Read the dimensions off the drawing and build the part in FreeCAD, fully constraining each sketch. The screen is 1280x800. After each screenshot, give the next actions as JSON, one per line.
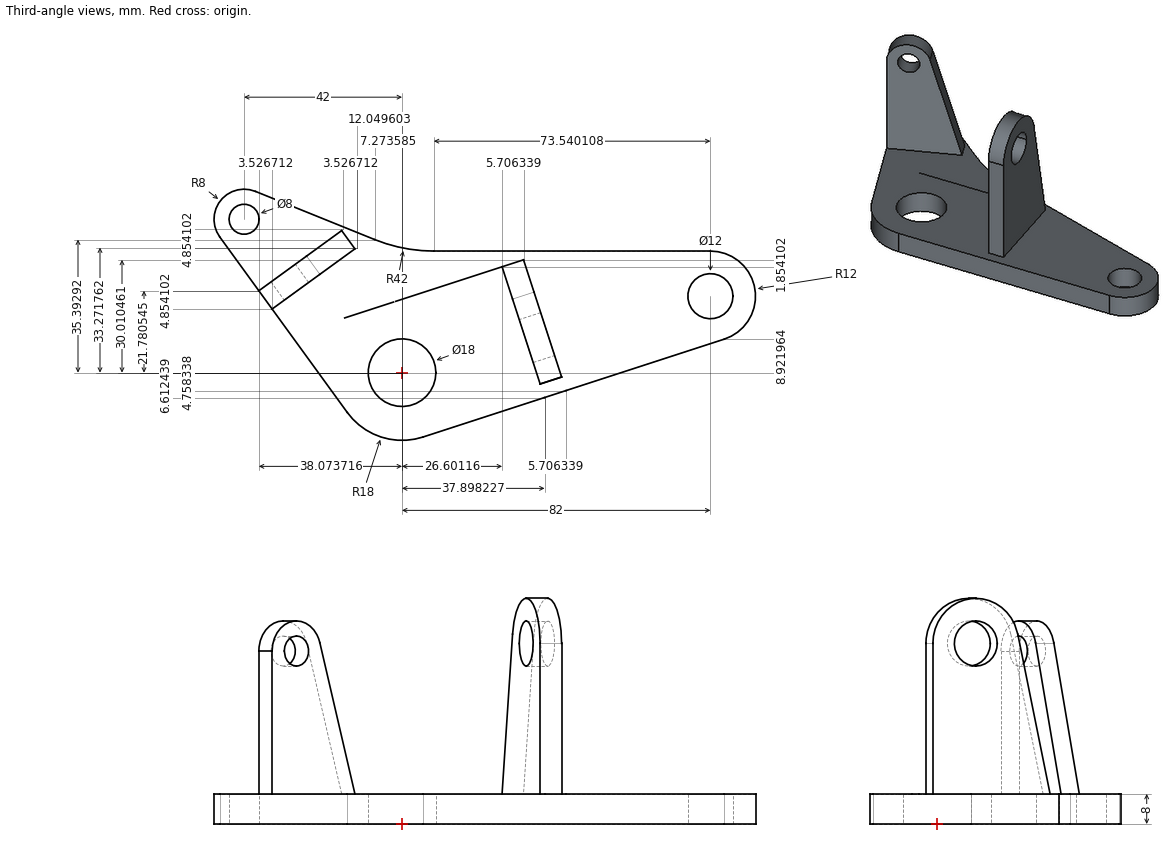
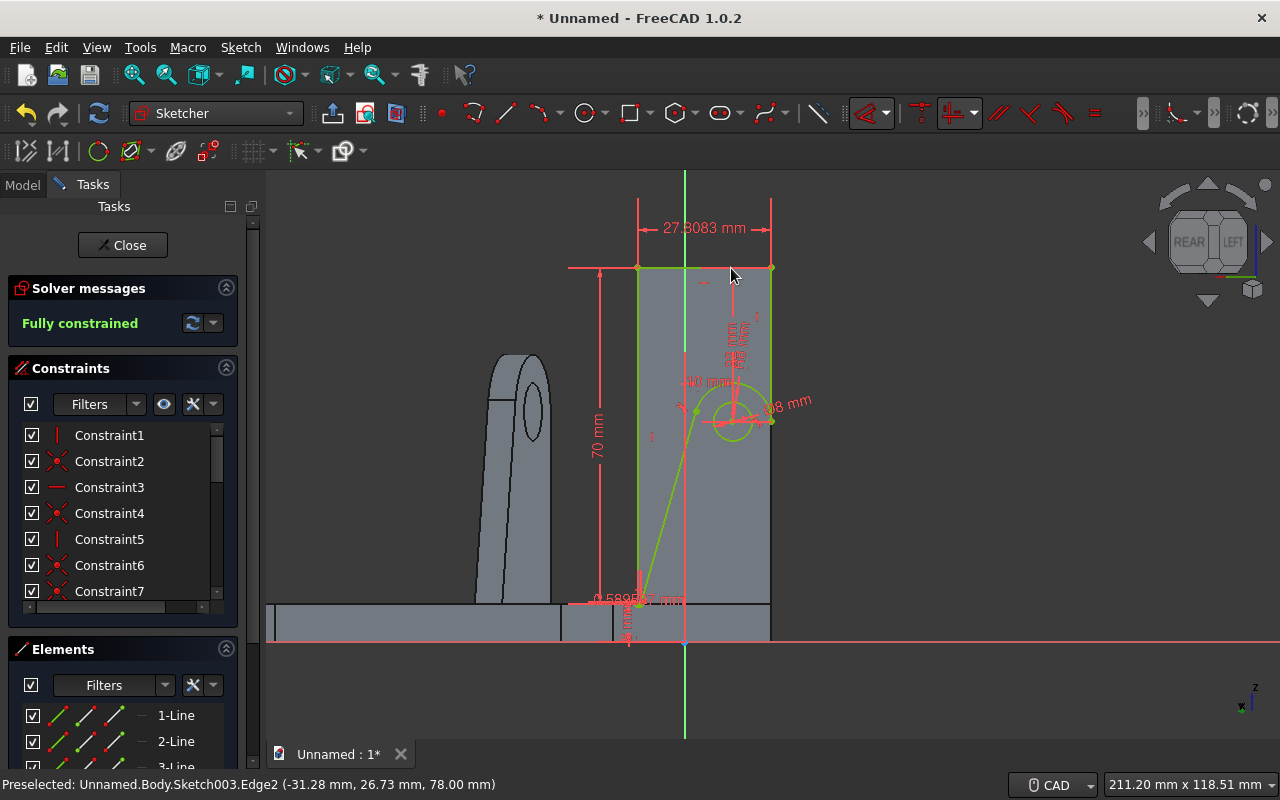
{"action": "left_click", "coordinate": [123, 245]}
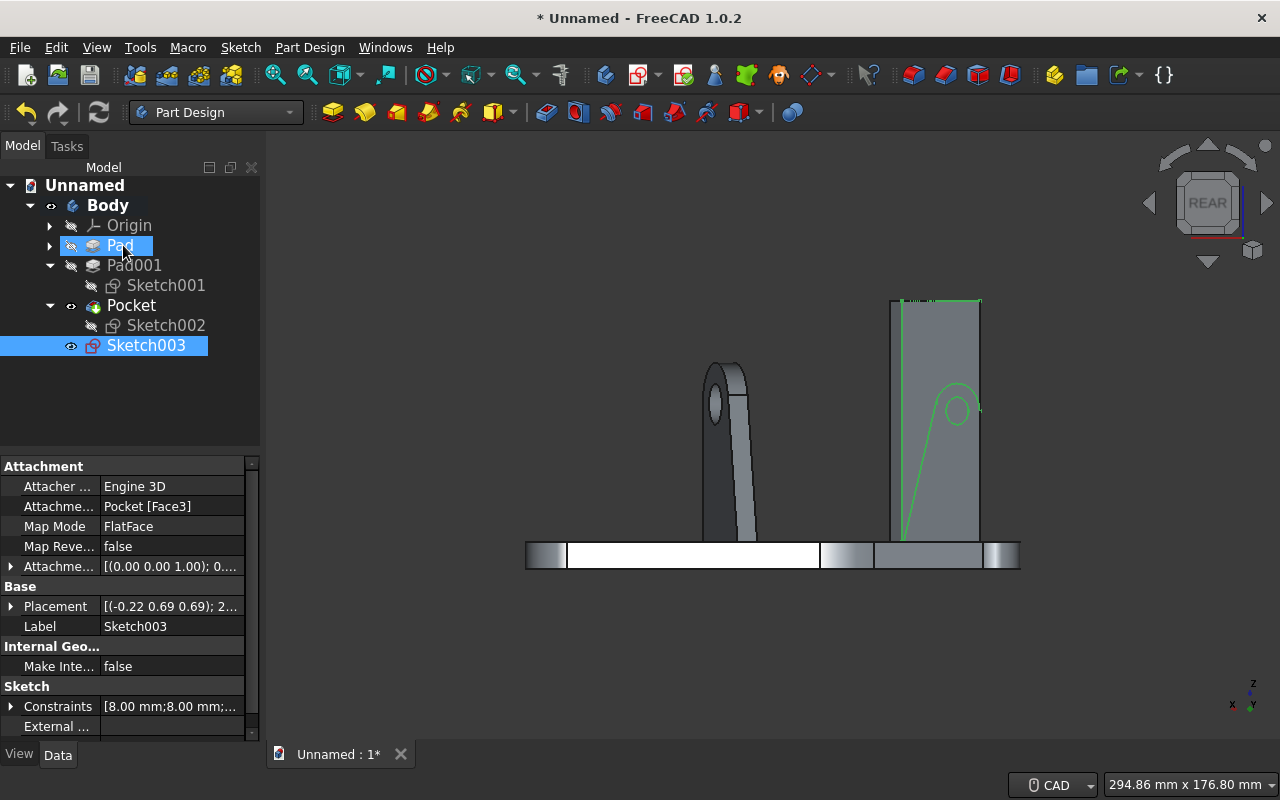
{"action": "left_click", "coordinate": [548, 112]}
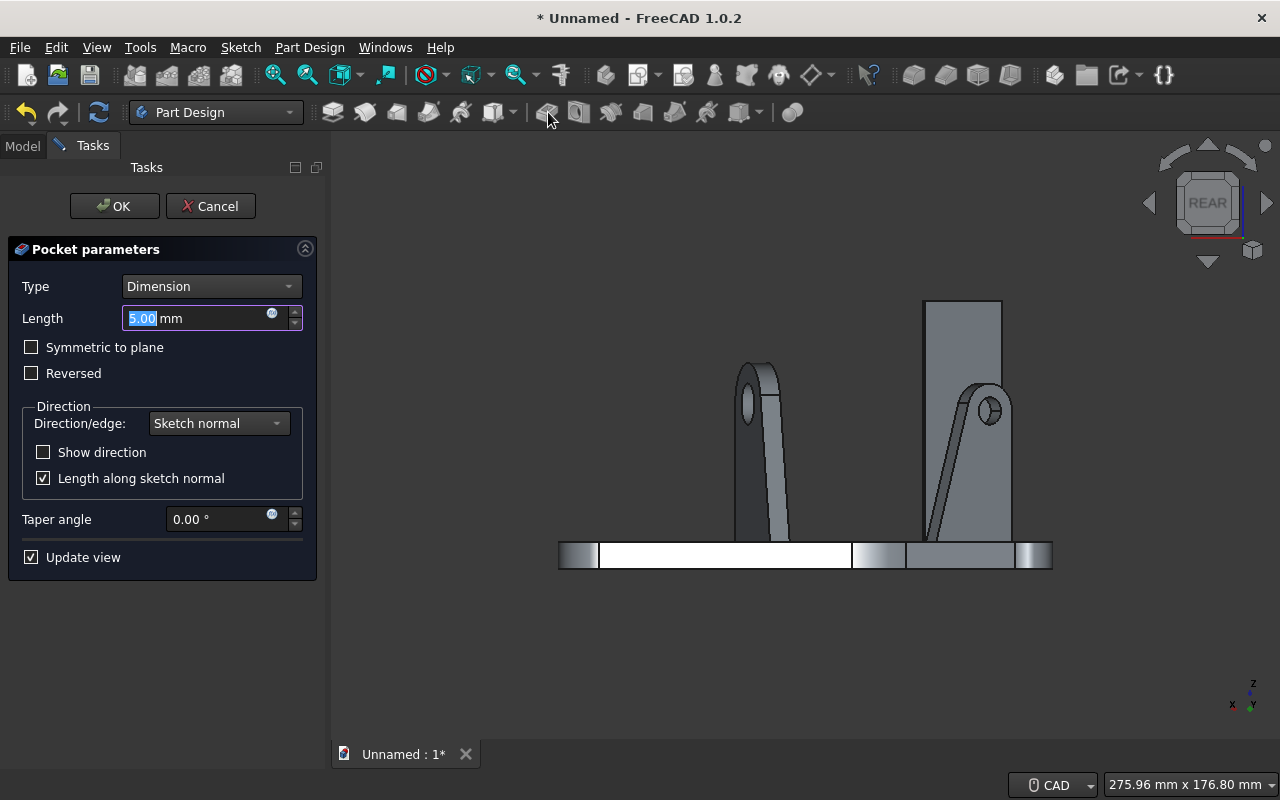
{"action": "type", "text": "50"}
{"action": "key", "text": "Tab"}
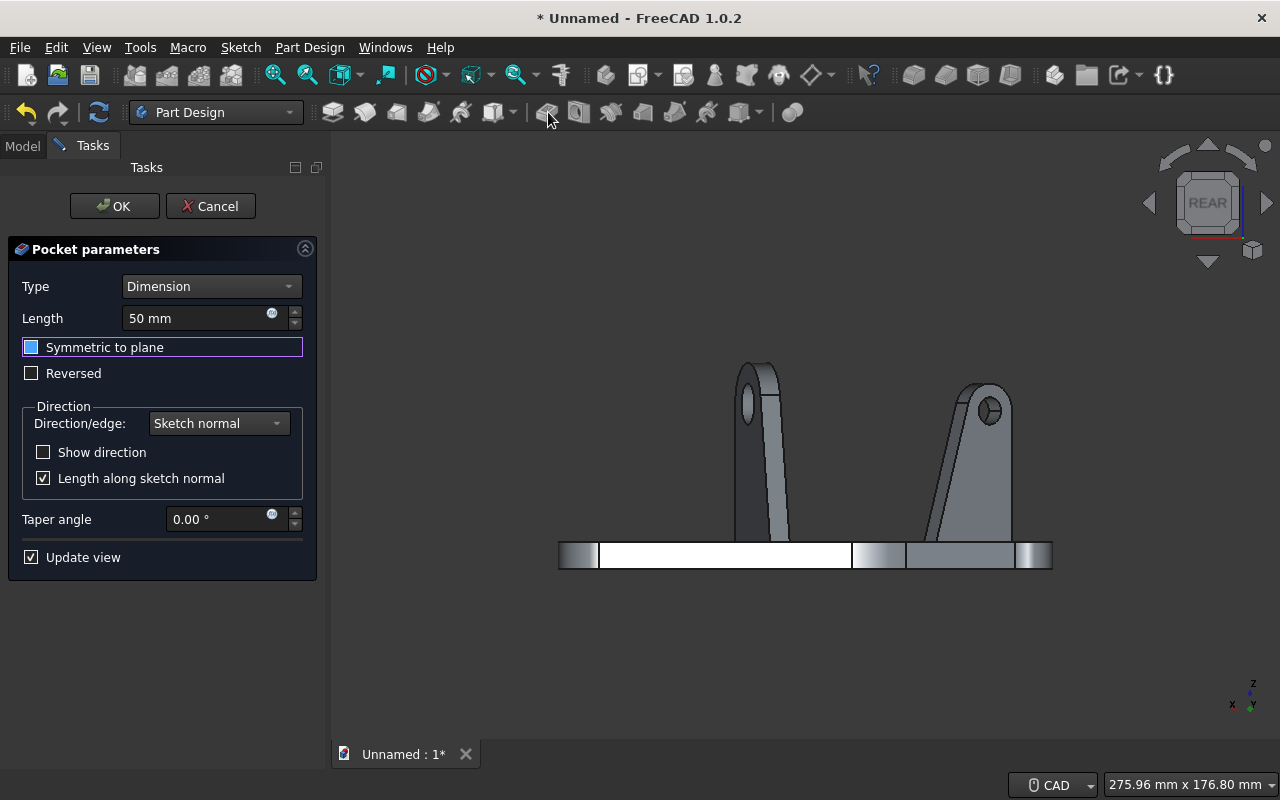
{"action": "left_click", "coordinate": [115, 206]}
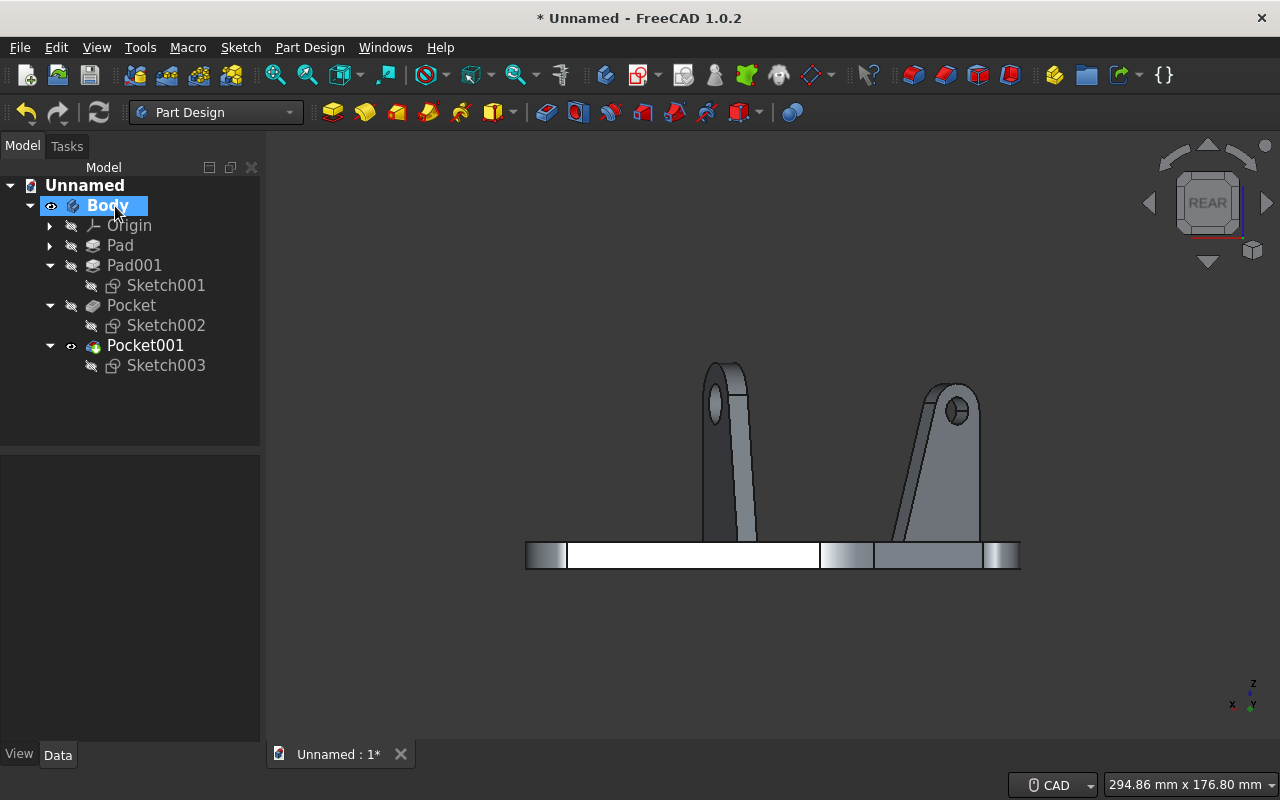
{"action": "key", "text": "0"}